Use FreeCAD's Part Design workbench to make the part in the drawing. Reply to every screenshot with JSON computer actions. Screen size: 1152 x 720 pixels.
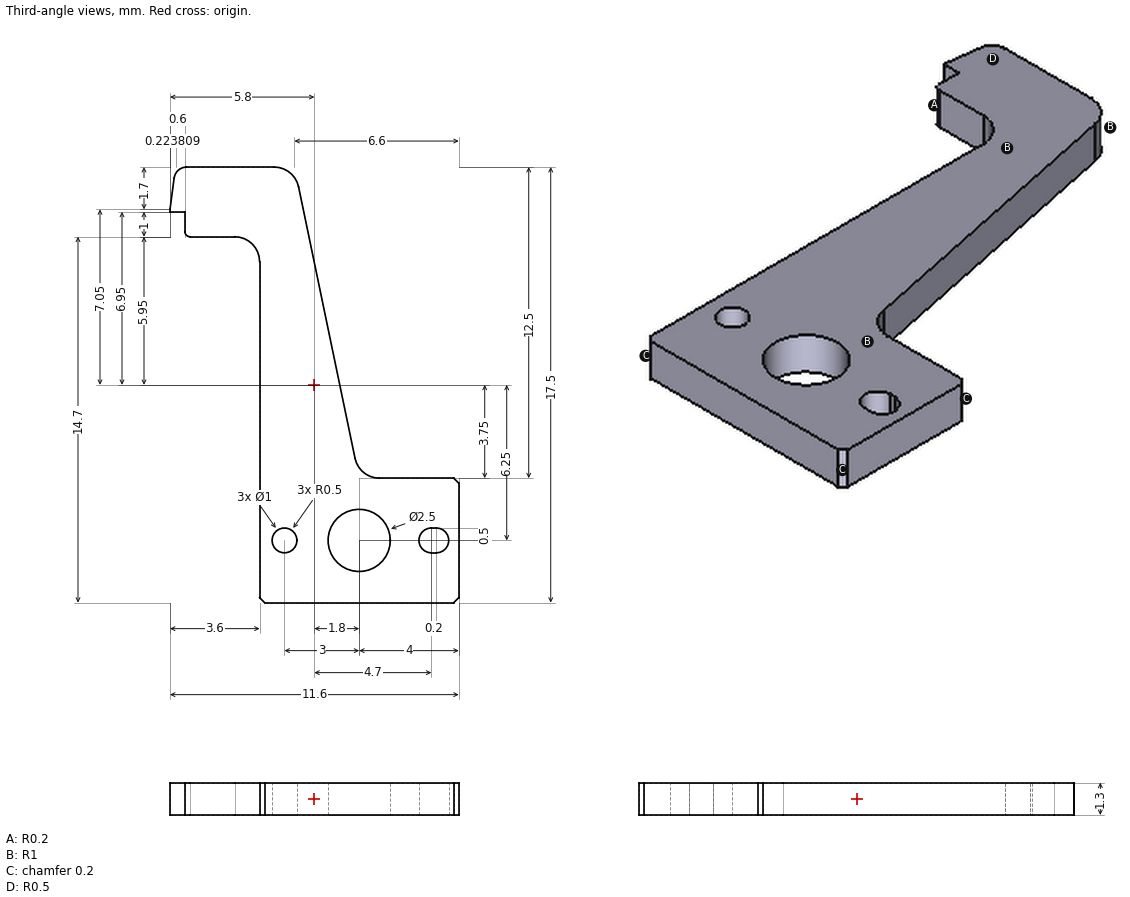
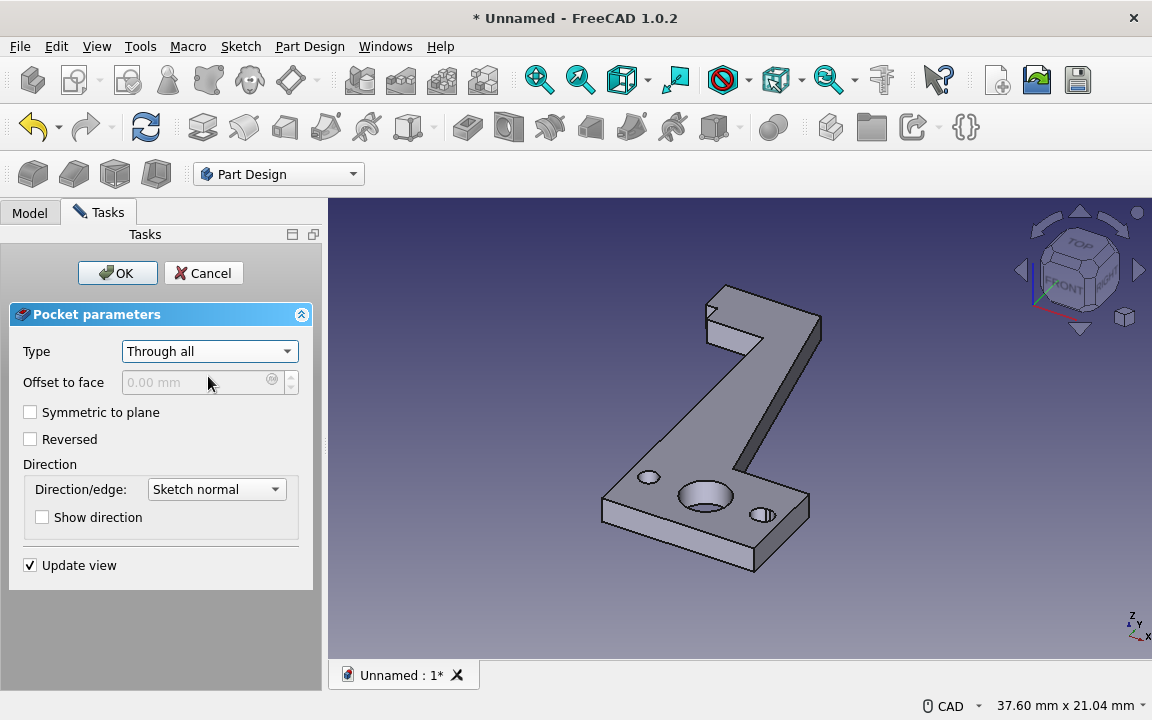
{"action": "left_click", "coordinate": [118, 273]}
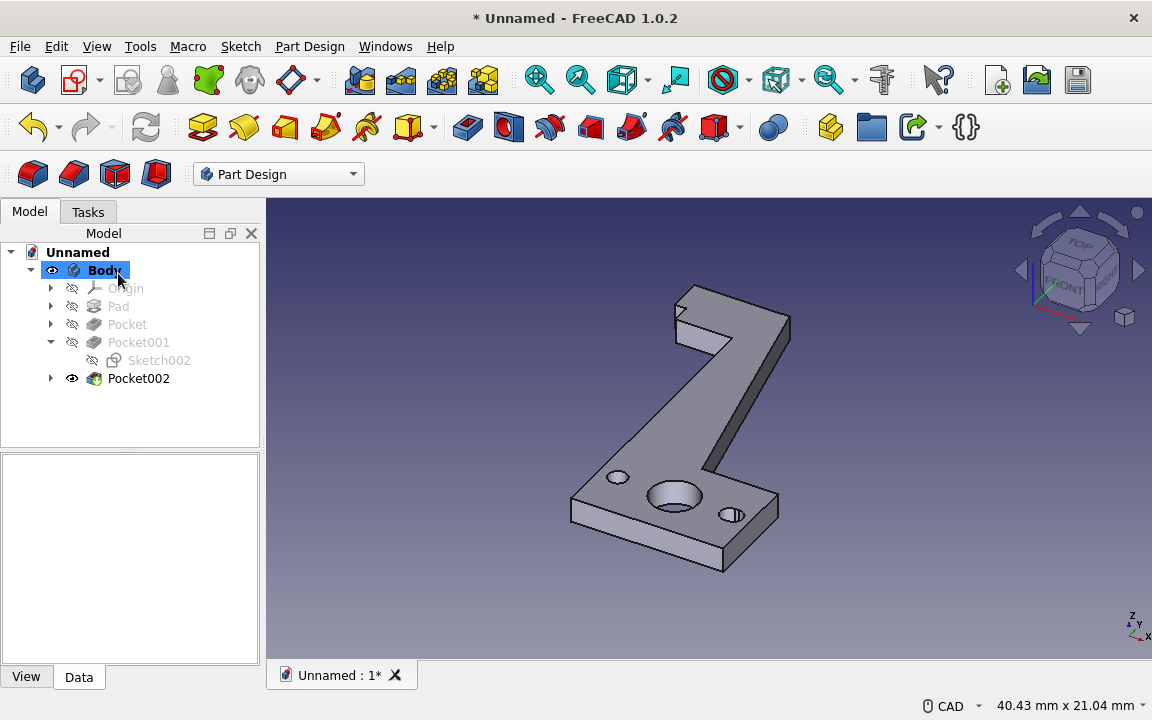
{"action": "key", "text": "0"}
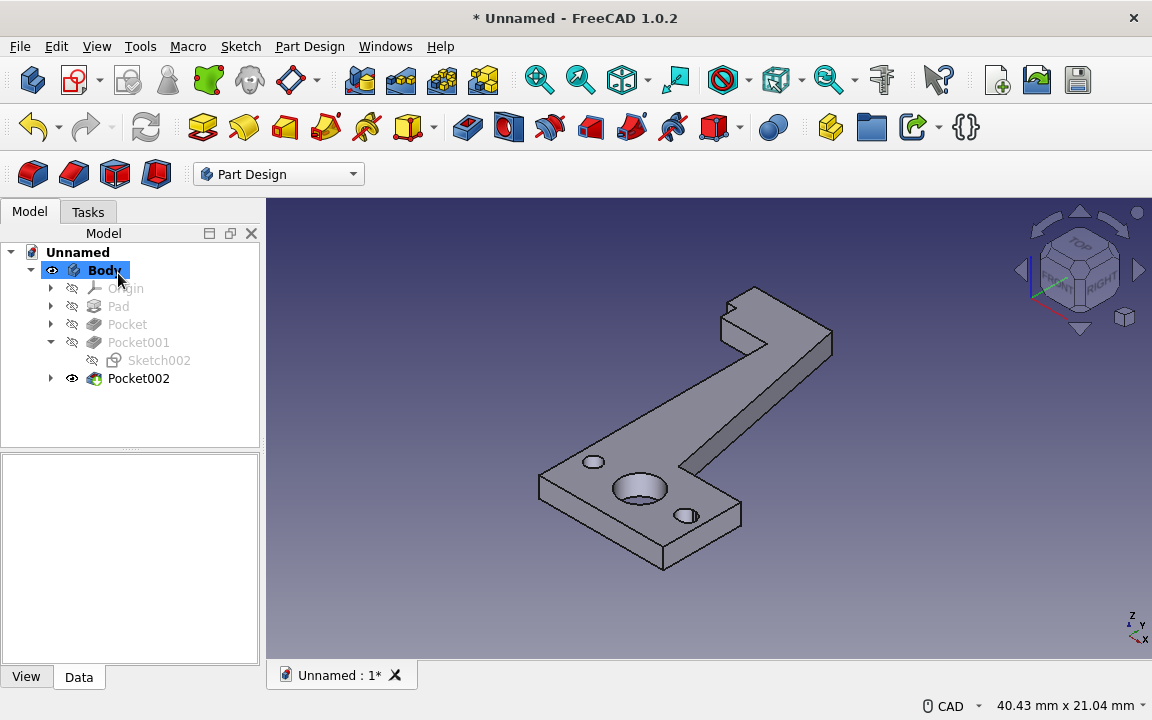
{"action": "key", "text": "2"}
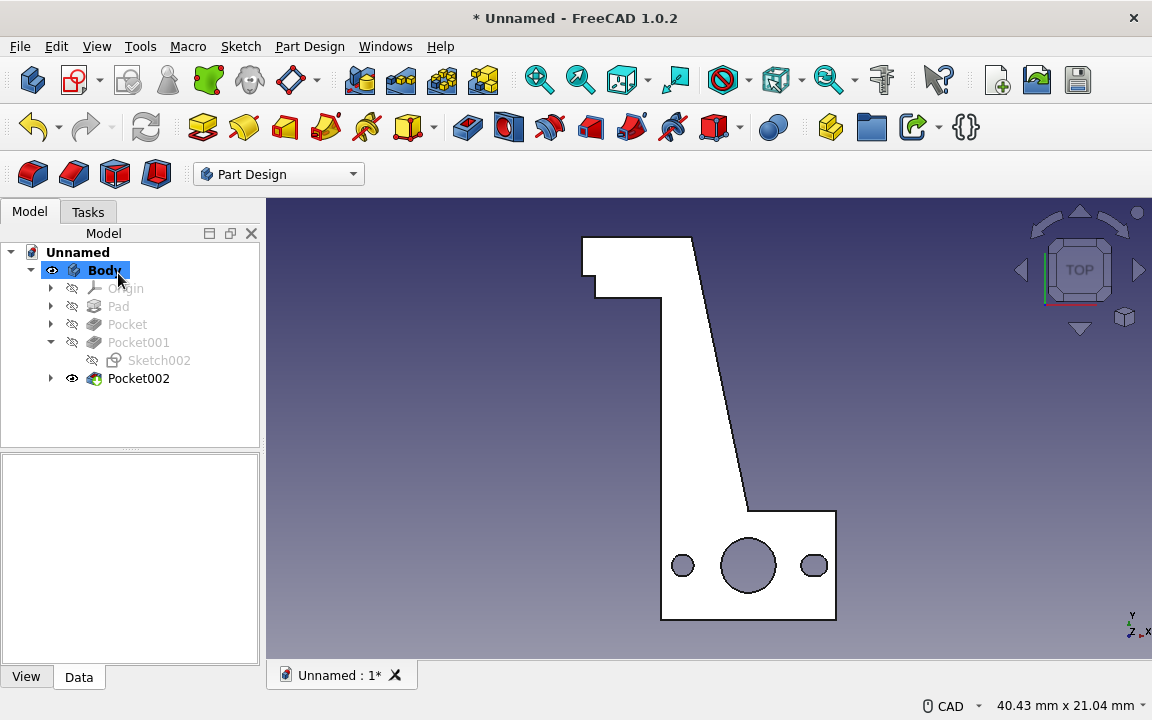
{"action": "key", "text": "1"}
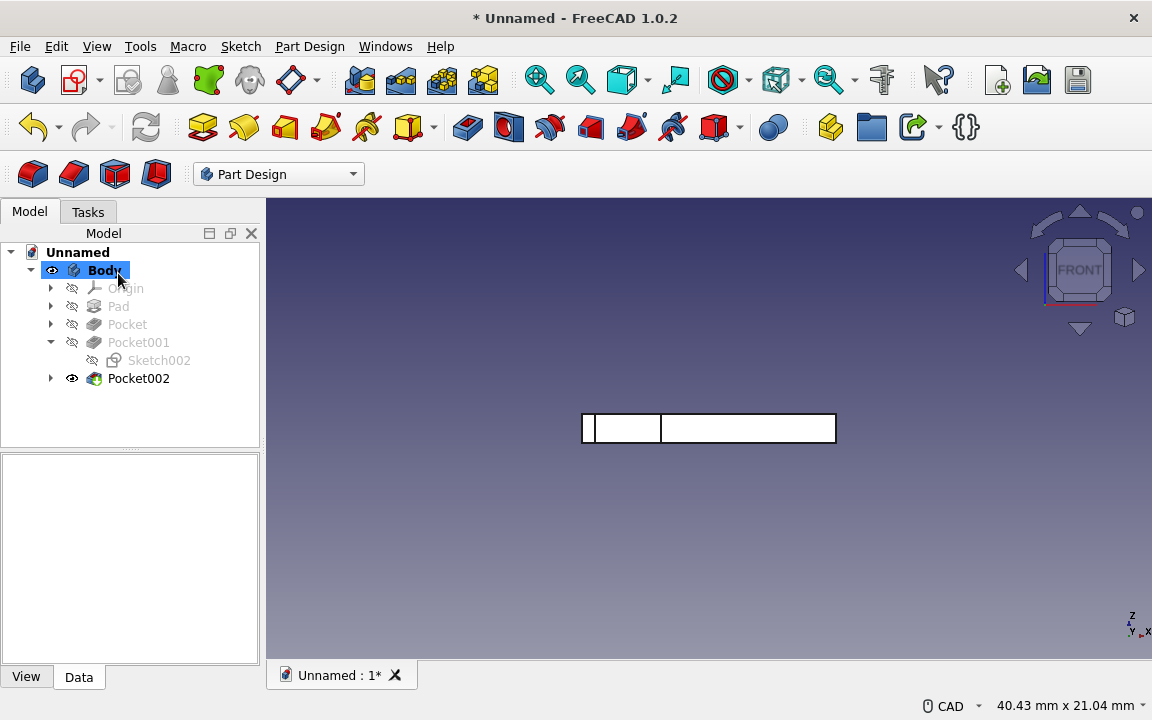
{"action": "left_click", "coordinate": [540, 80]}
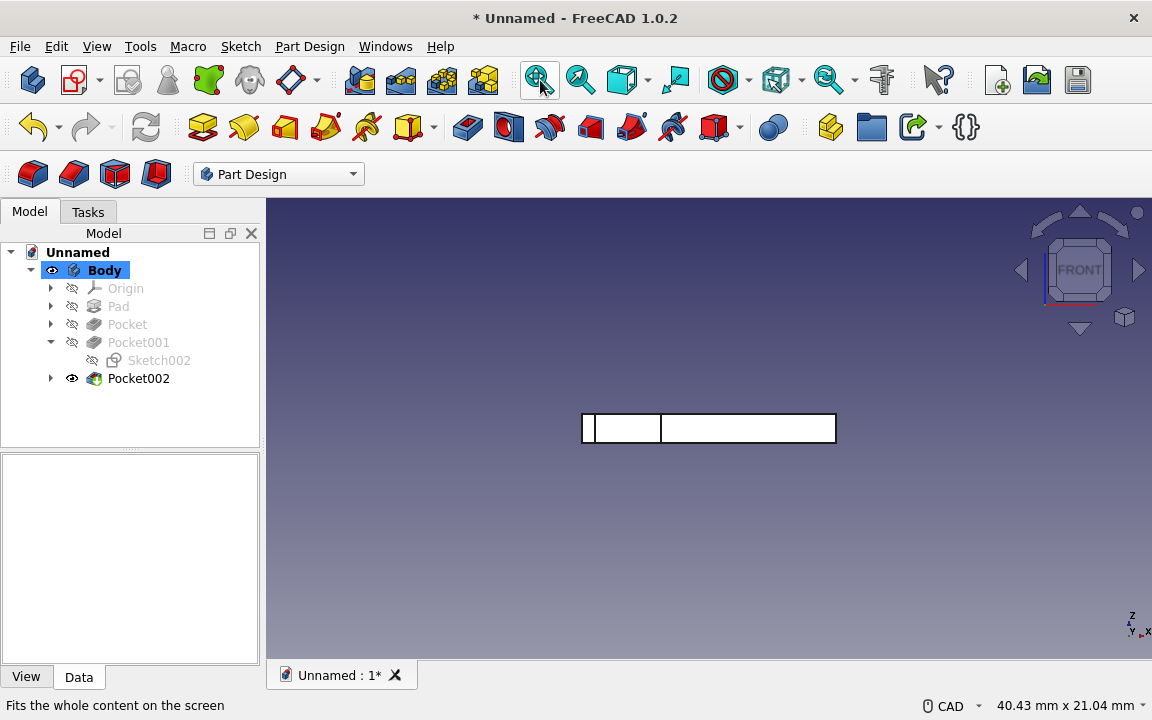
{"action": "left_click", "coordinate": [595, 428]}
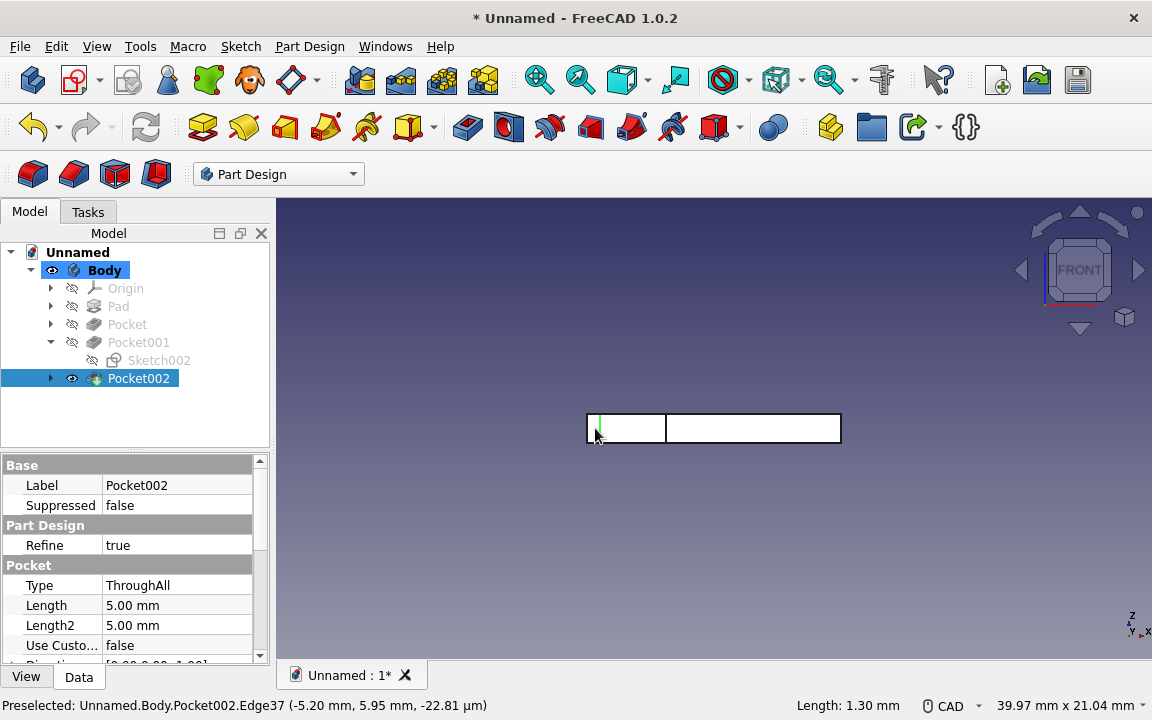
{"action": "left_click", "coordinate": [33, 174]}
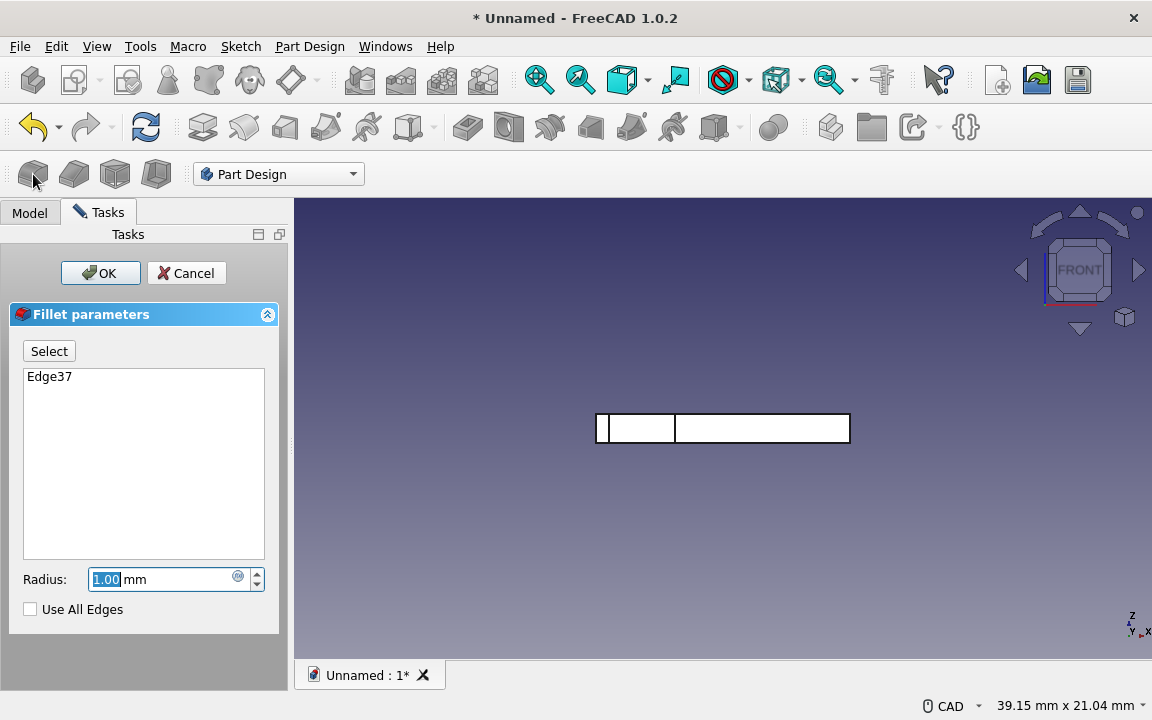
{"action": "type", "text": "0.2"}
{"action": "key", "text": "Tab"}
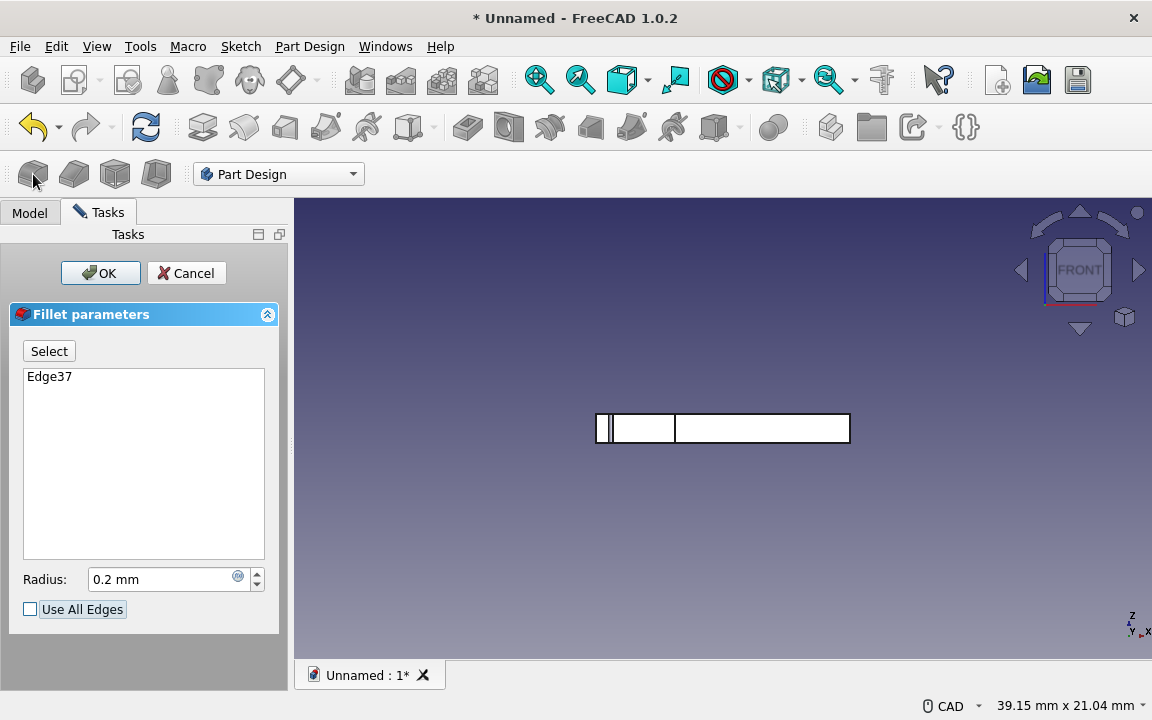
{"action": "left_click", "coordinate": [101, 273]}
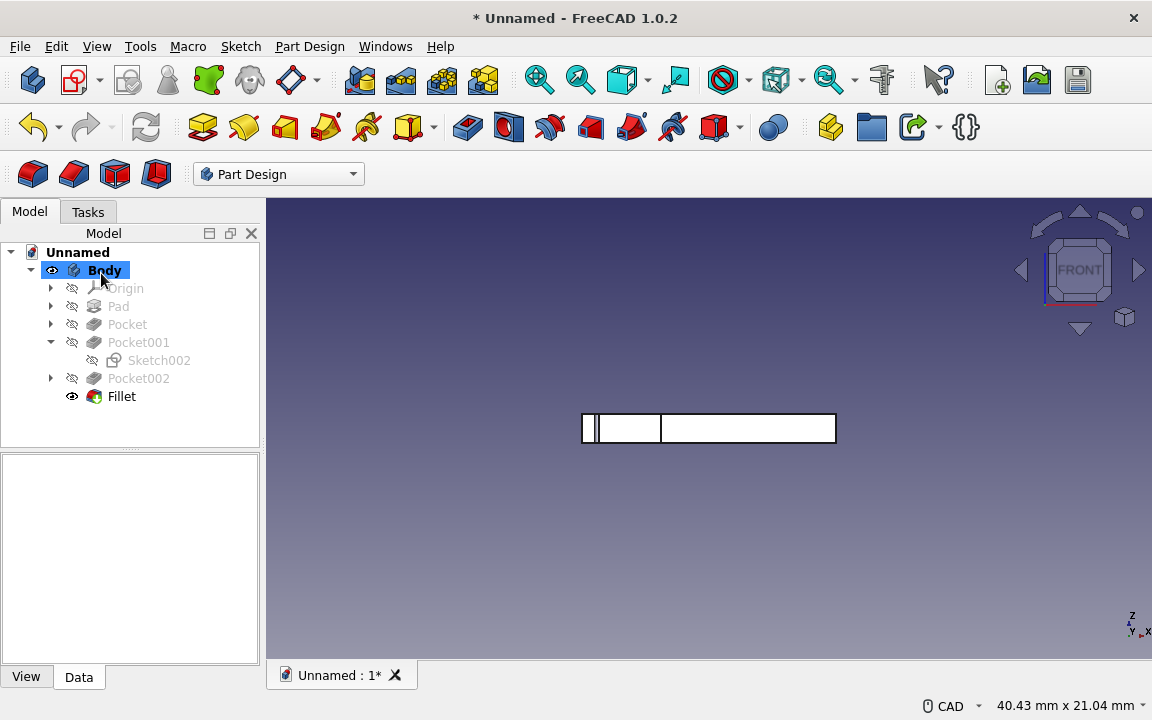
{"action": "left_click", "coordinate": [540, 80]}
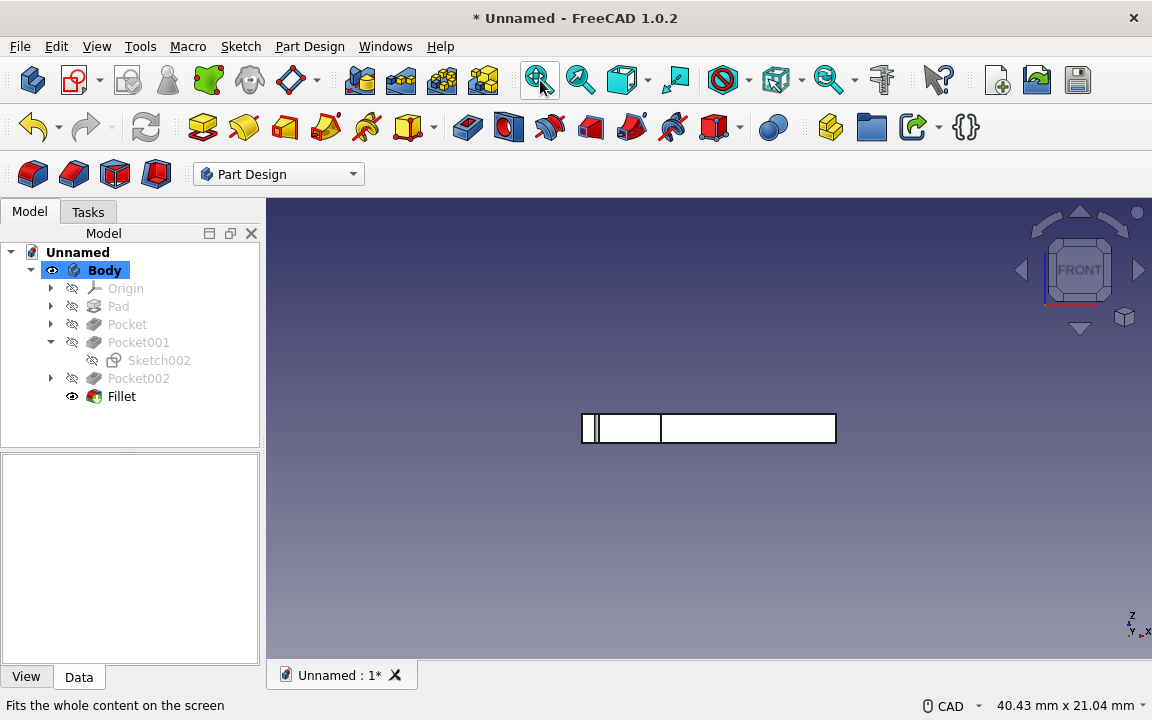
{"action": "key", "text": "0"}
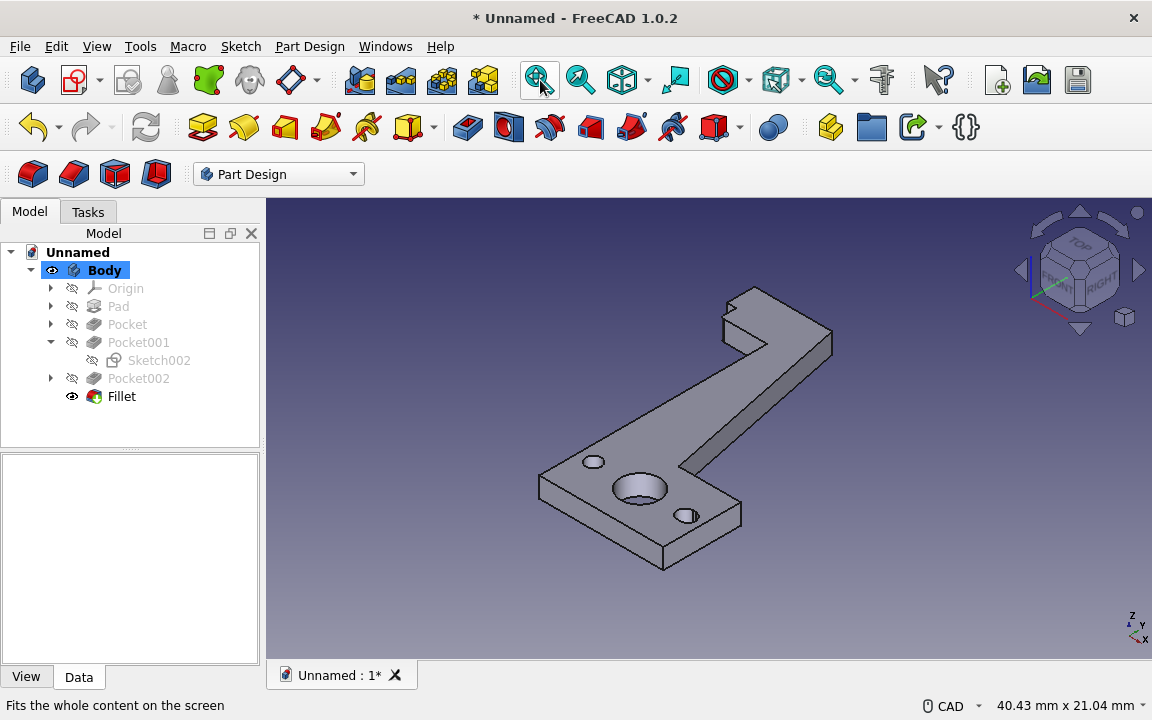
{"action": "left_click", "coordinate": [670, 438]}